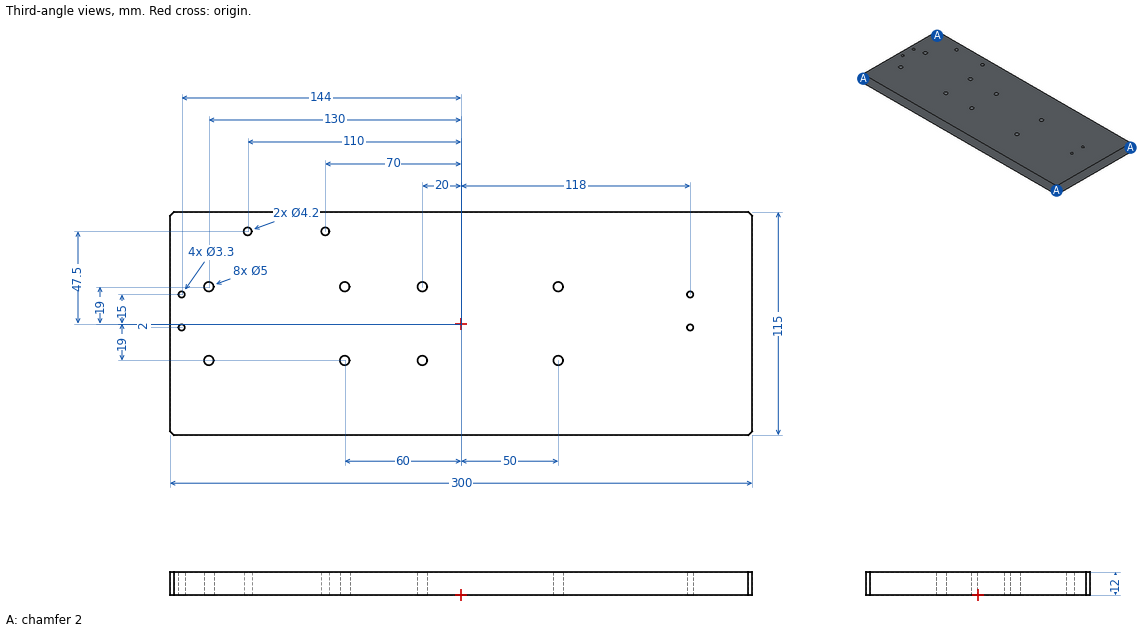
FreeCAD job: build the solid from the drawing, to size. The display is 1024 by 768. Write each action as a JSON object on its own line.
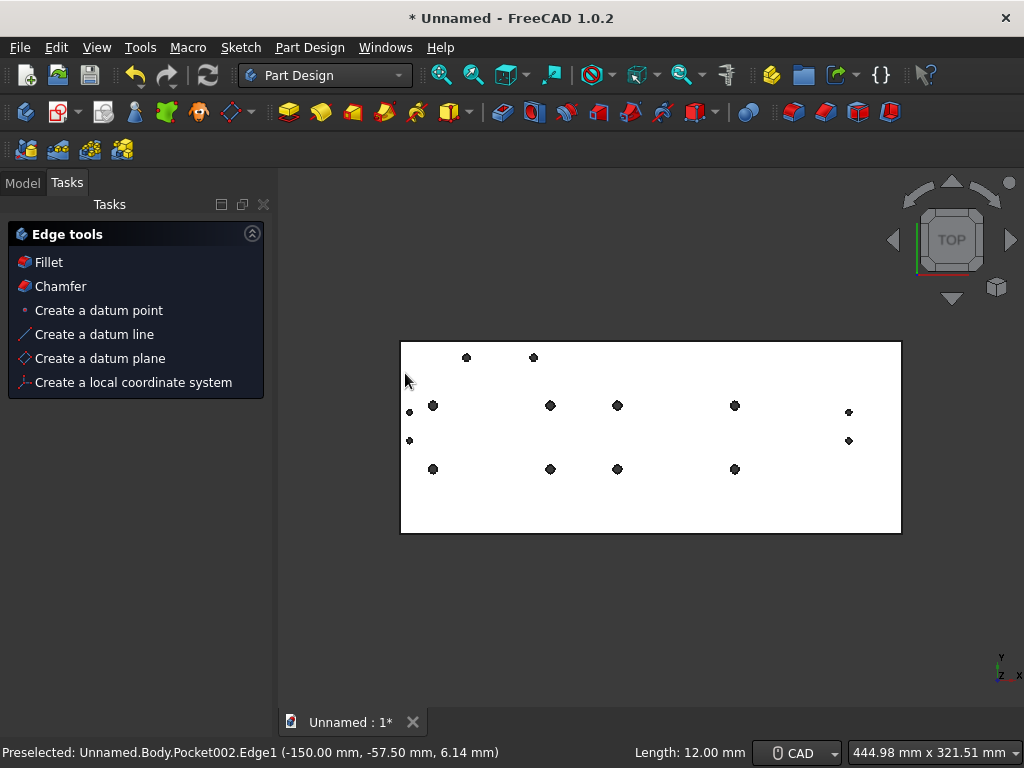
{"action": "scroll", "coordinate": [400, 533], "scroll_direction": "up", "scroll_amount": 4}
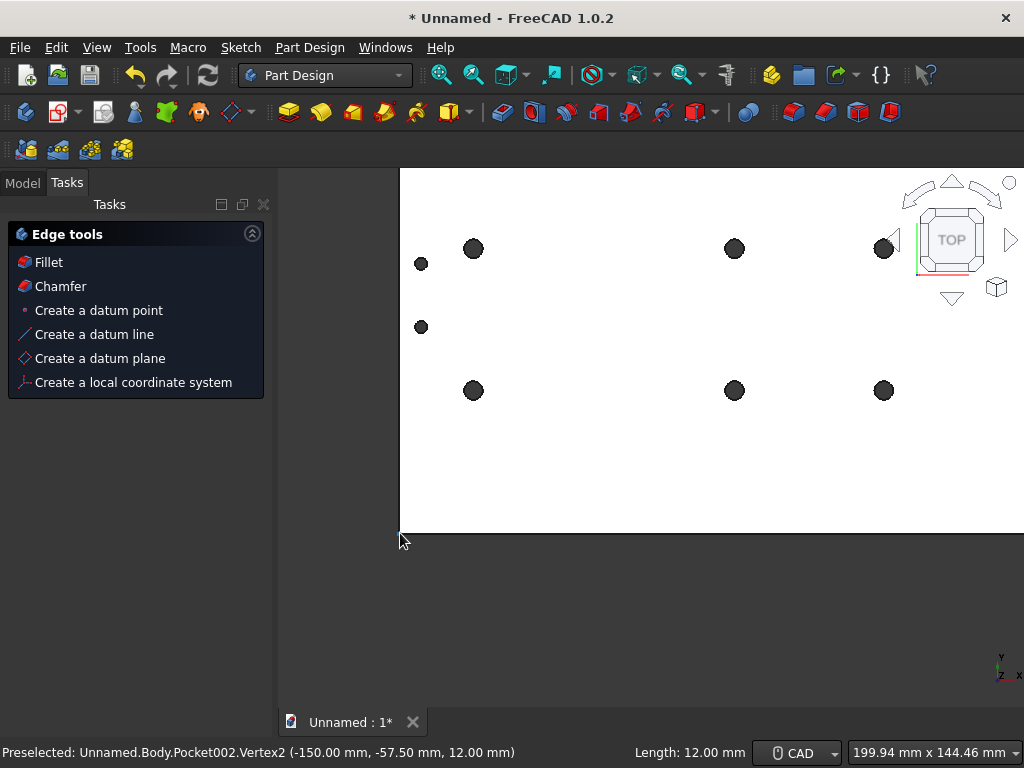
{"action": "key", "text": "v f"}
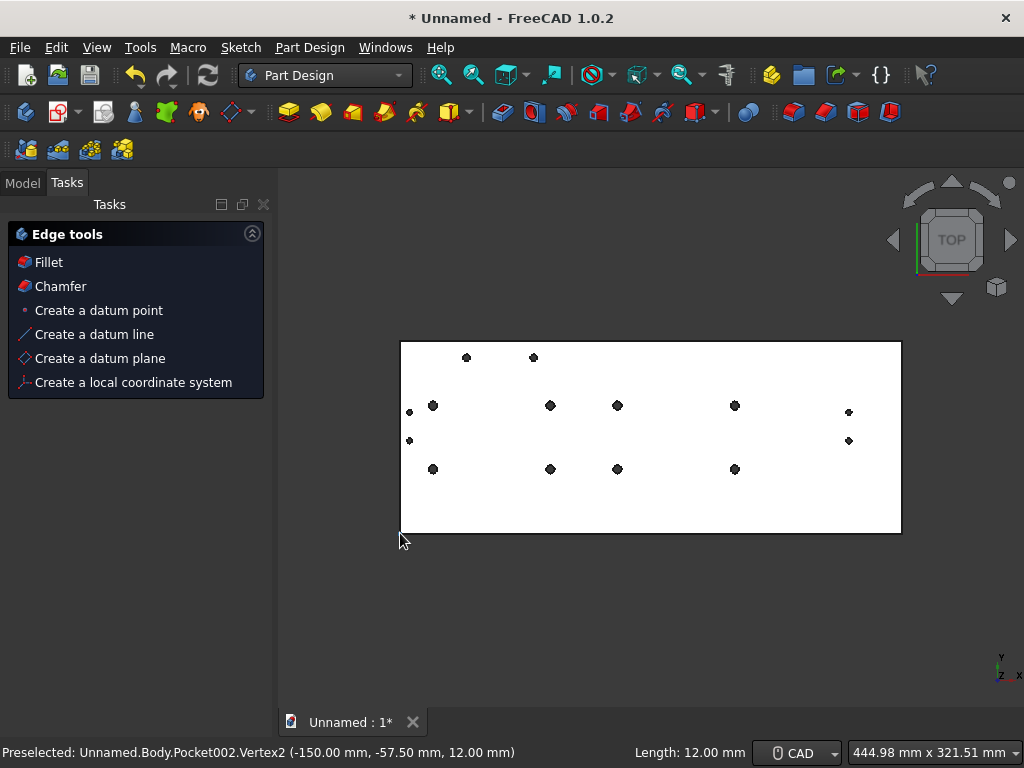
{"action": "key", "text": "1"}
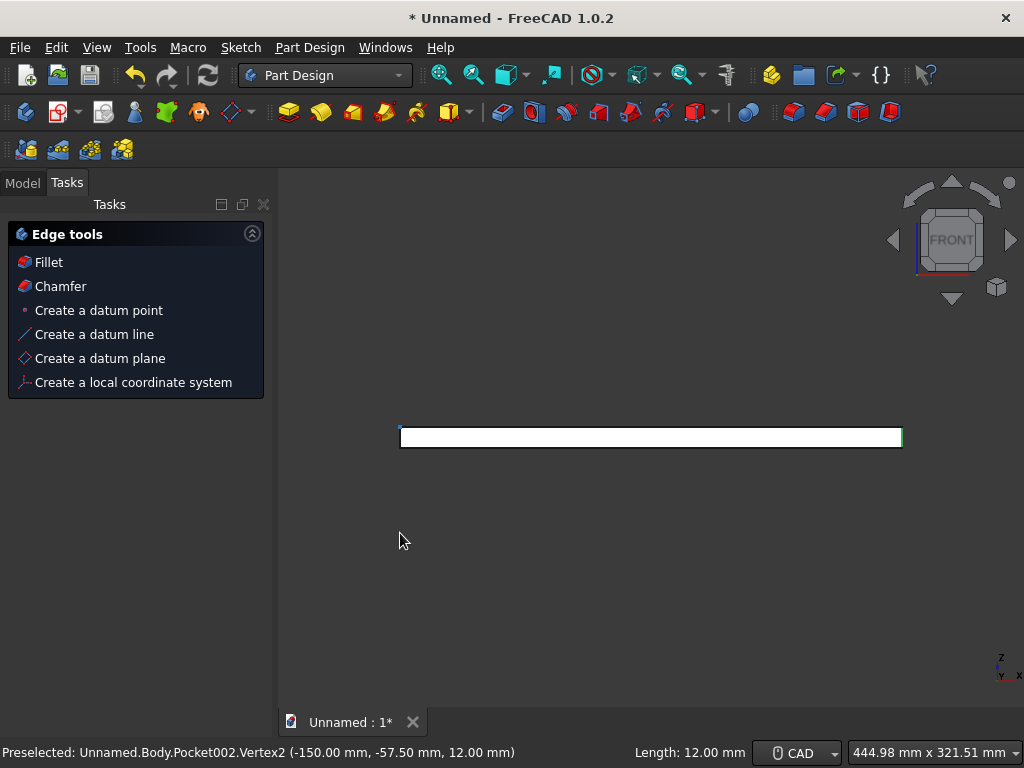
{"action": "left_click", "coordinate": [400, 436], "text": "ctrl"}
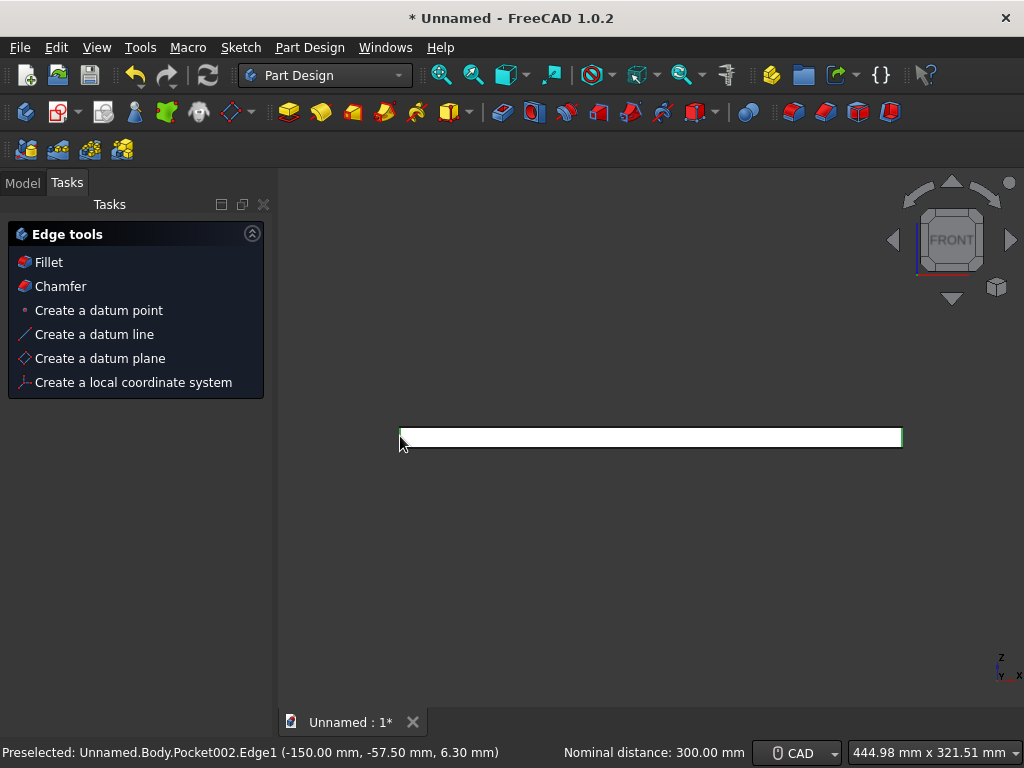
{"action": "scroll", "coordinate": [400, 436], "scroll_direction": "up", "scroll_amount": 4}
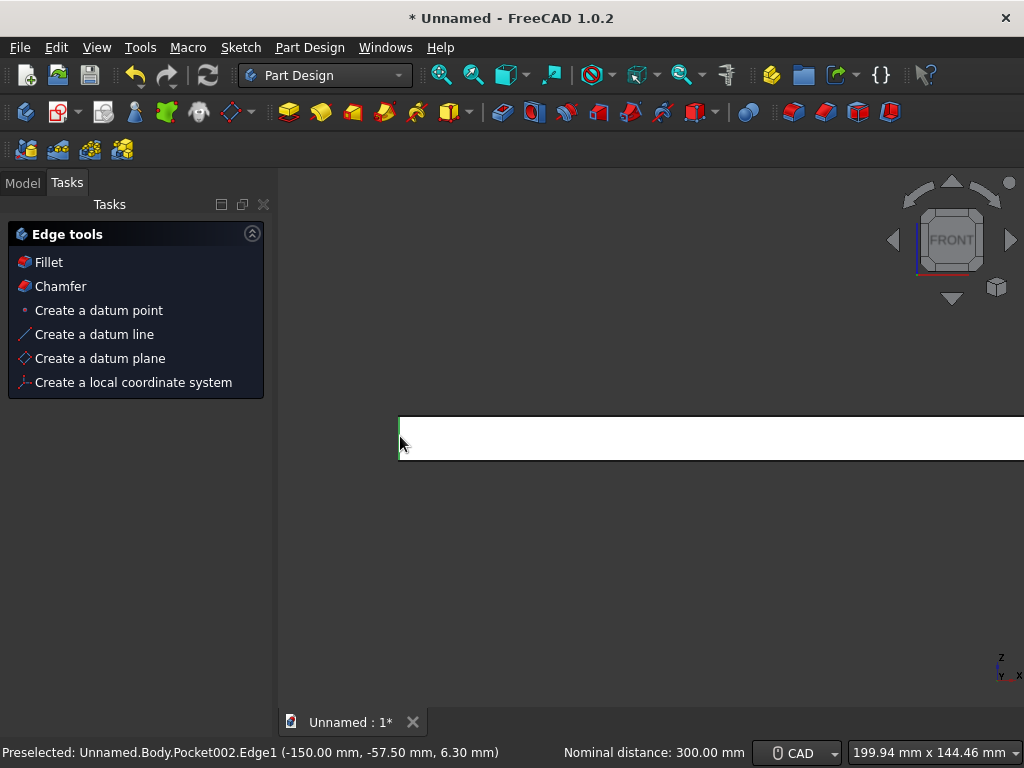
{"action": "key", "text": "v f"}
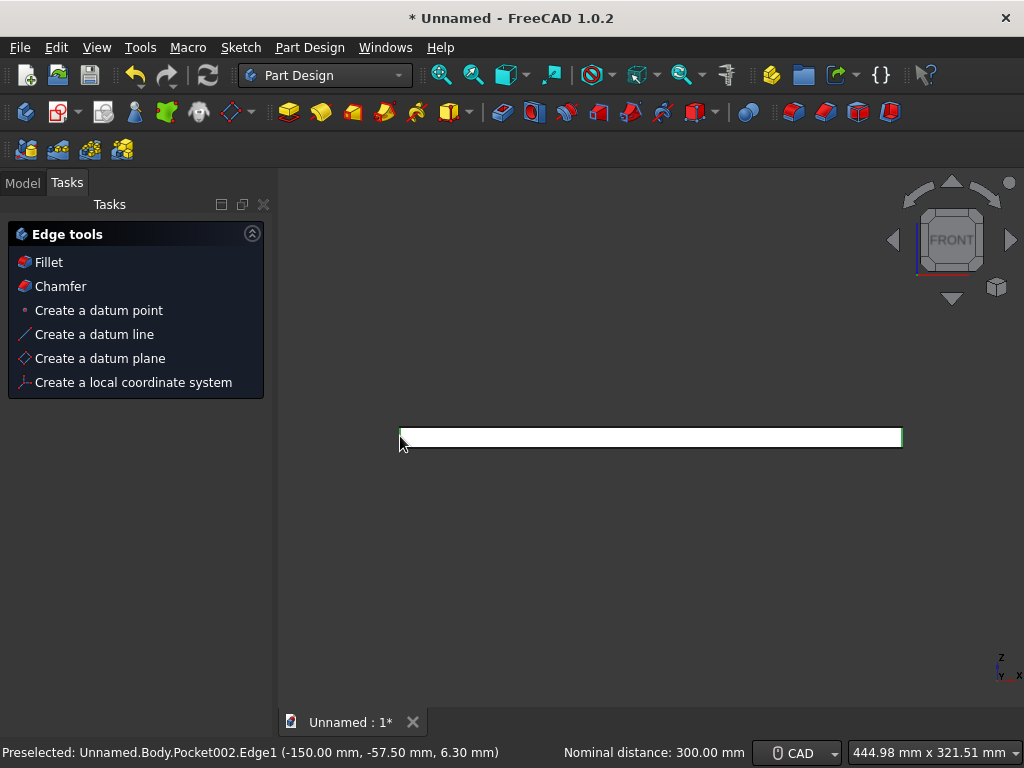
{"action": "key", "text": "3"}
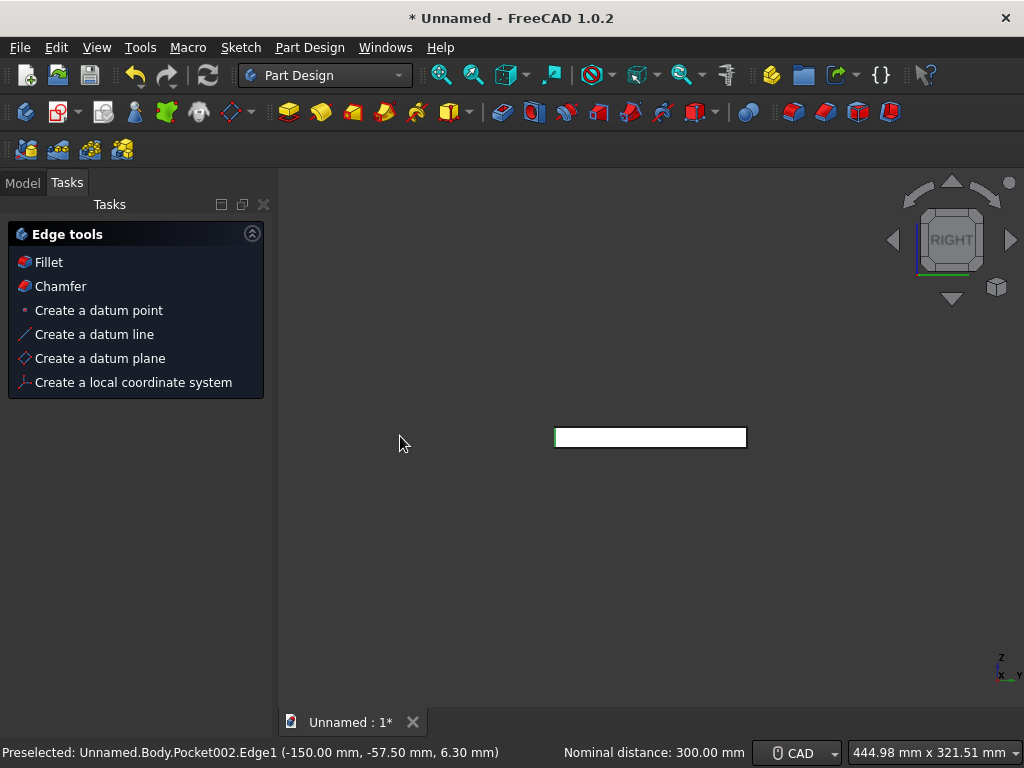
{"action": "left_click", "coordinate": [442, 76]}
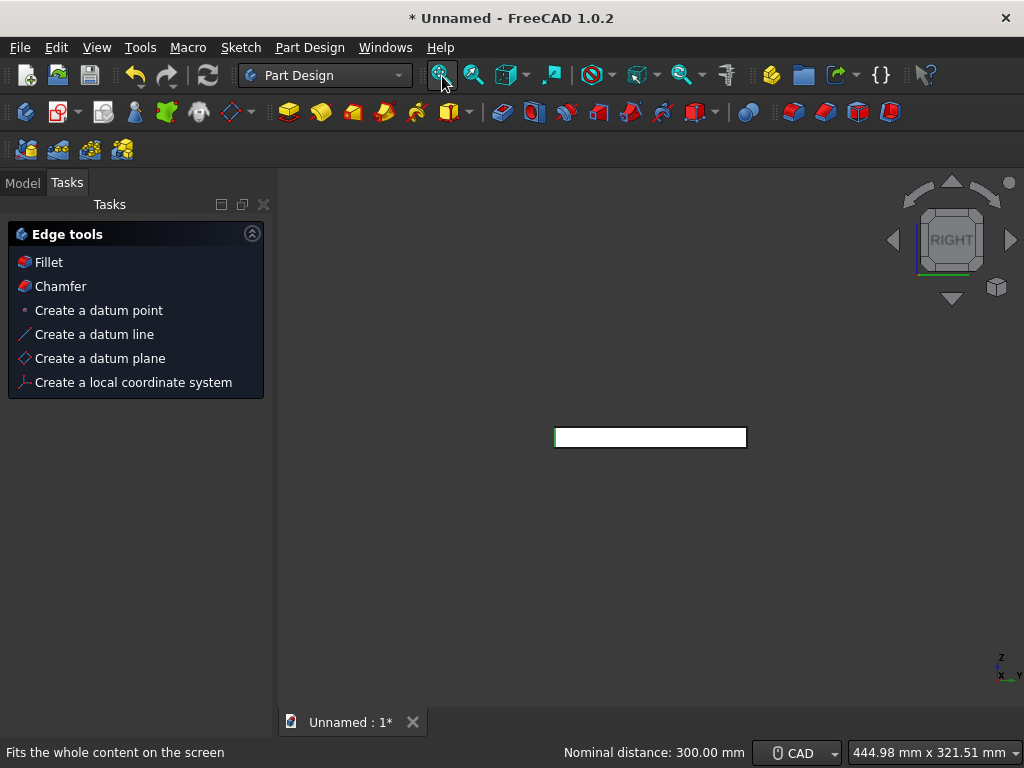
{"action": "left_click", "coordinate": [747, 436], "text": "ctrl"}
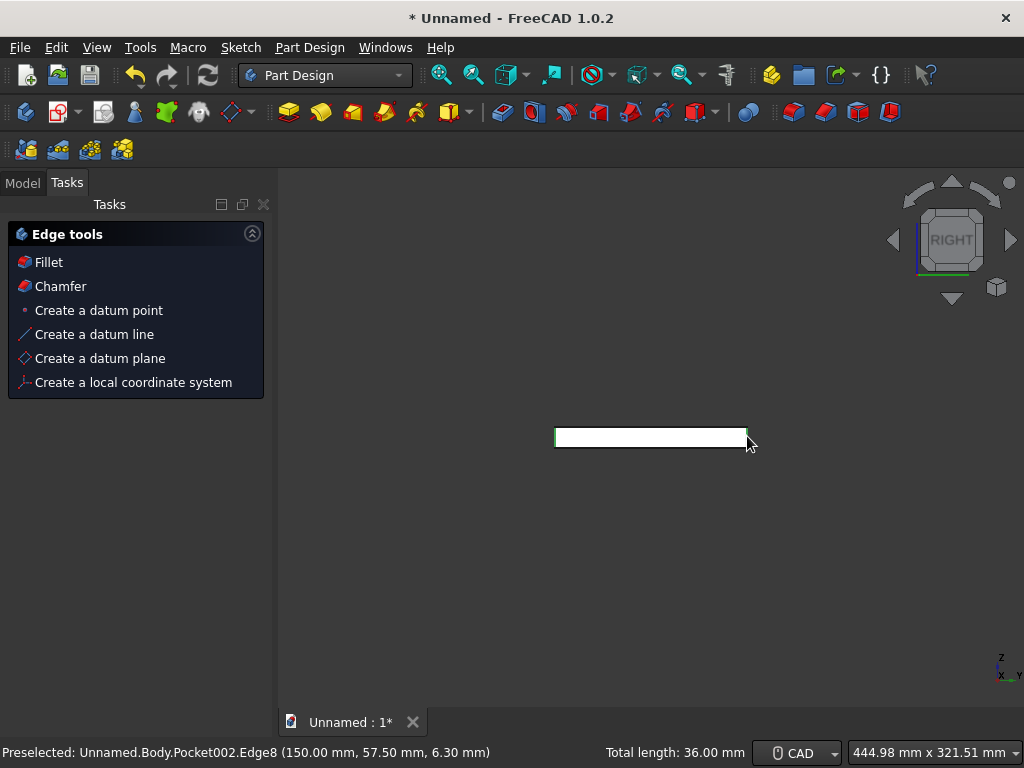
{"action": "scroll", "coordinate": [747, 436], "scroll_direction": "up", "scroll_amount": 4}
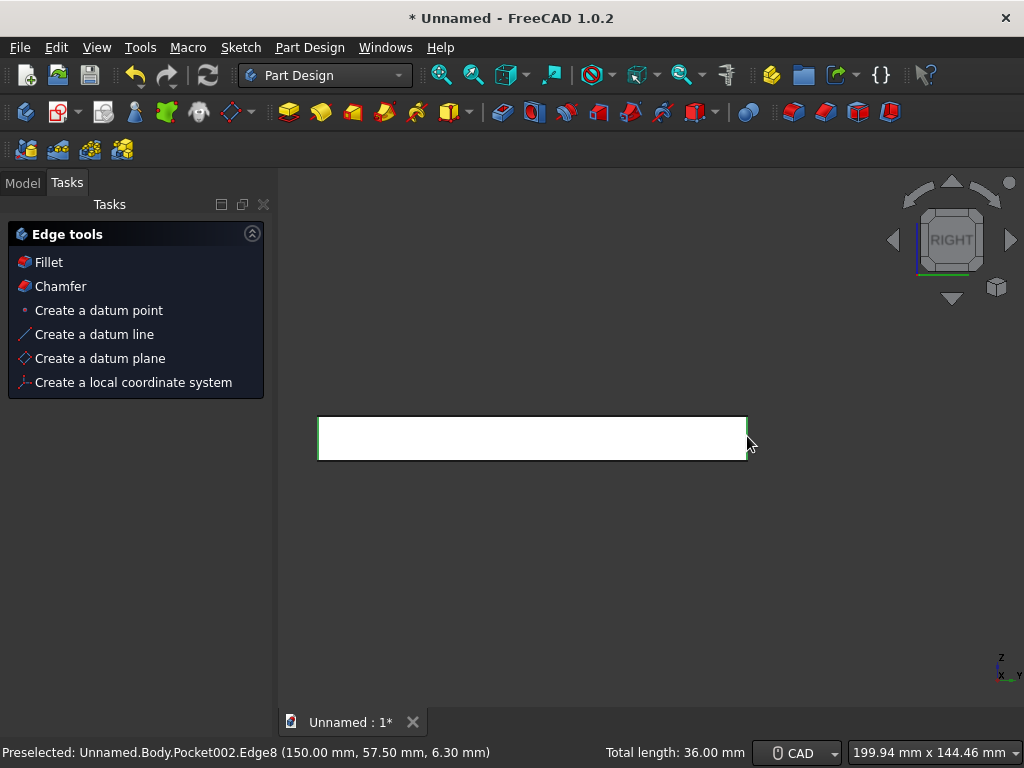
{"action": "left_click", "coordinate": [442, 76]}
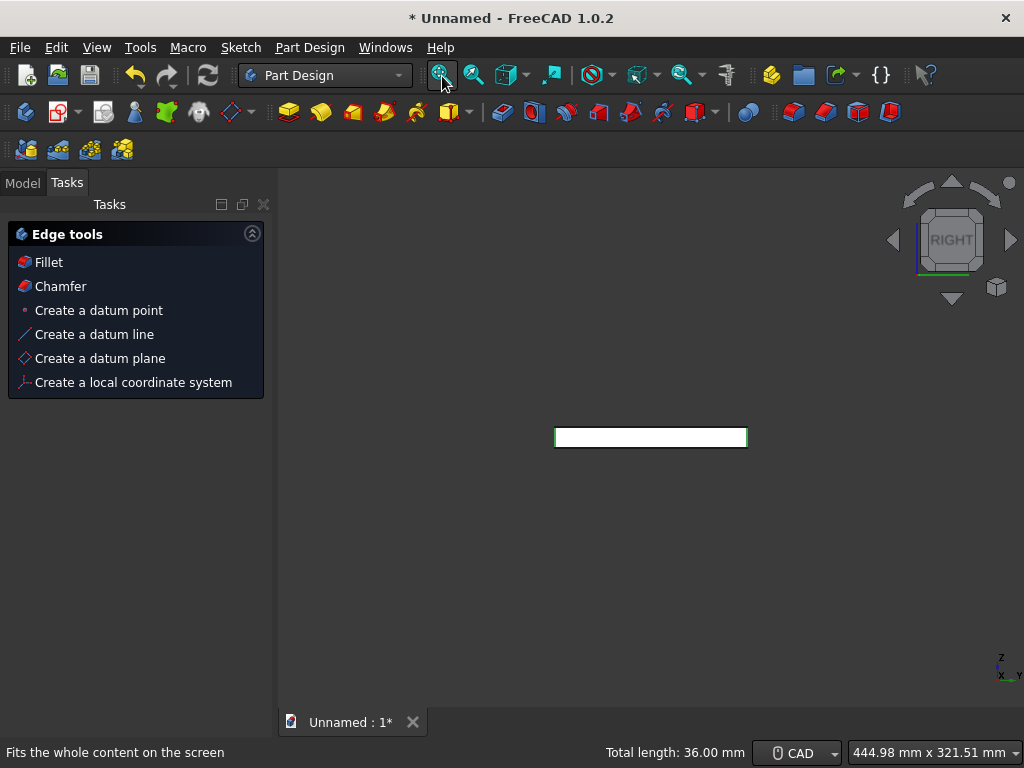
{"action": "key", "text": "5"}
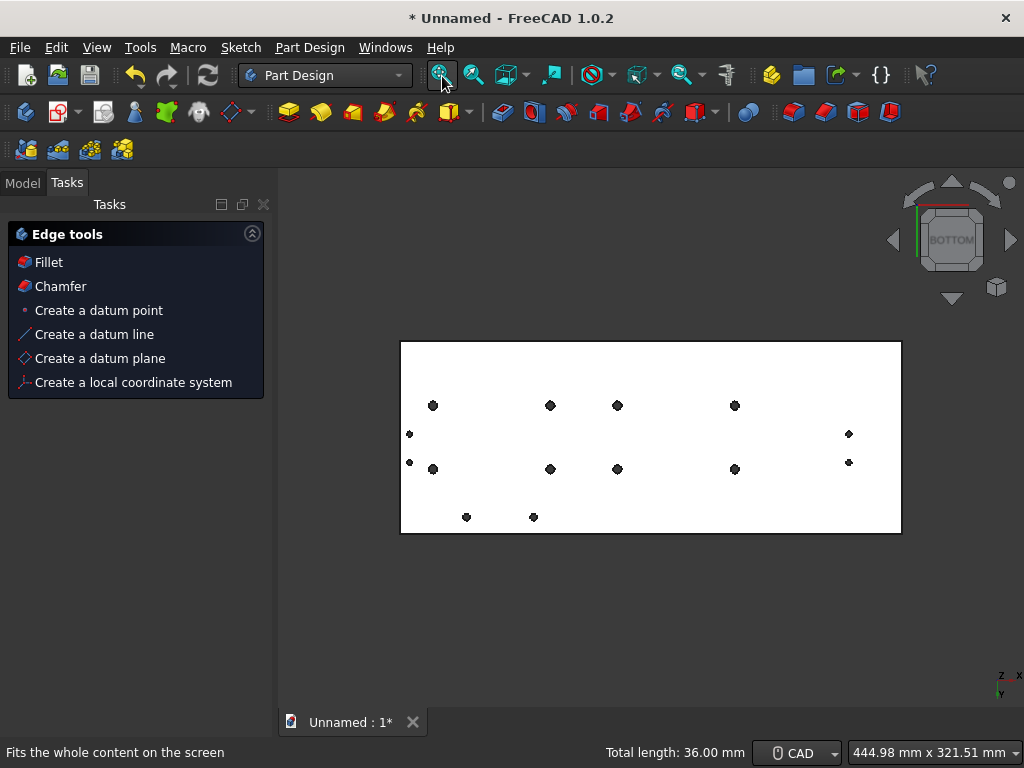
{"action": "scroll", "coordinate": [400, 533], "scroll_direction": "up", "scroll_amount": 4}